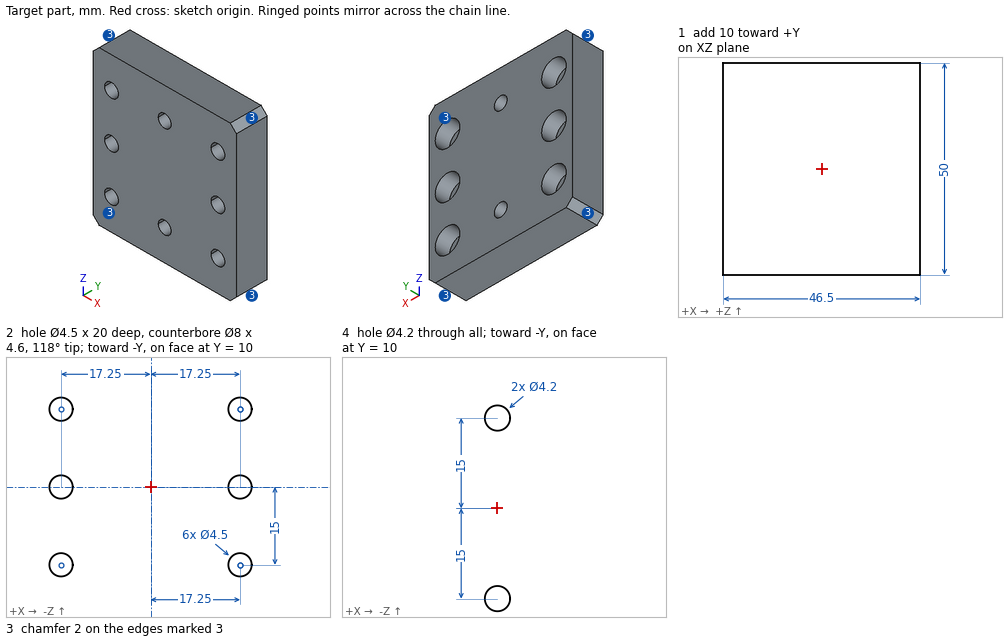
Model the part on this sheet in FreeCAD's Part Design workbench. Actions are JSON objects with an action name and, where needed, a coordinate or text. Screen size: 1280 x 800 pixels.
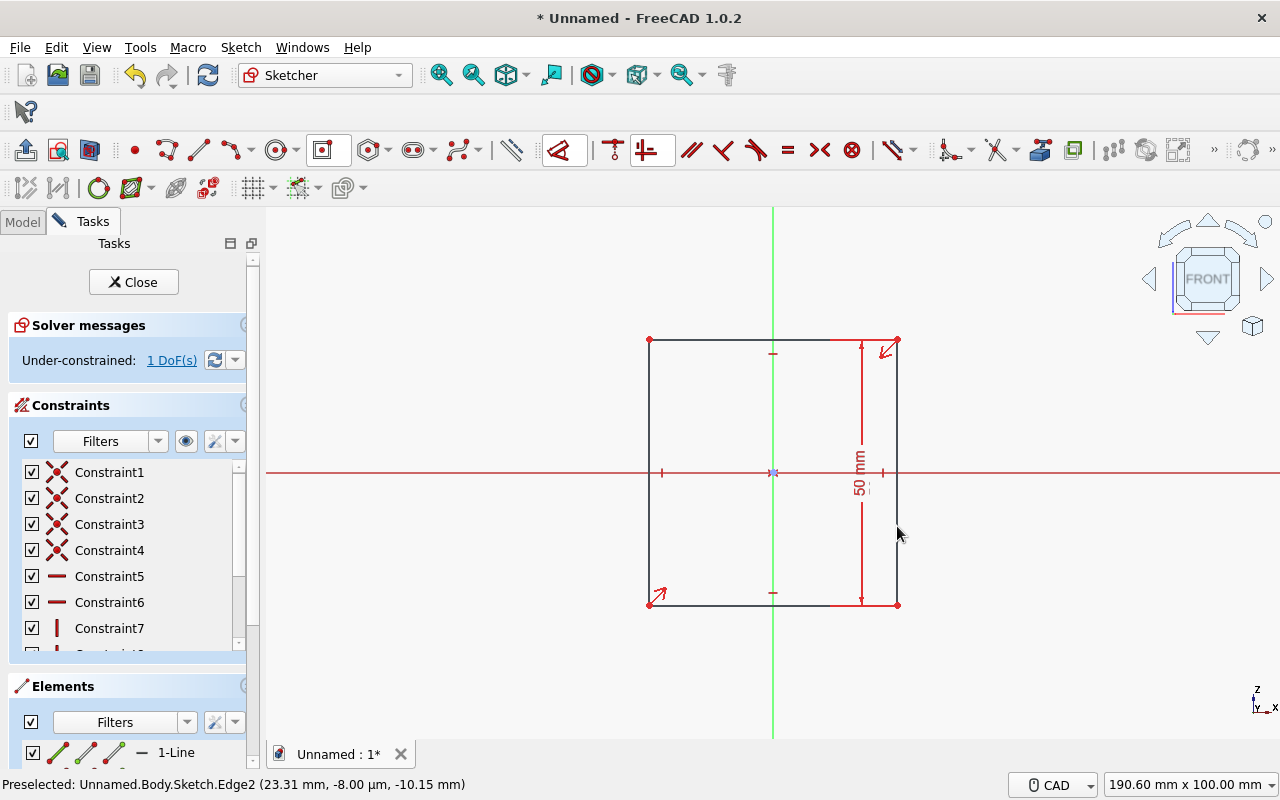
{"action": "left_click", "coordinate": [723, 606]}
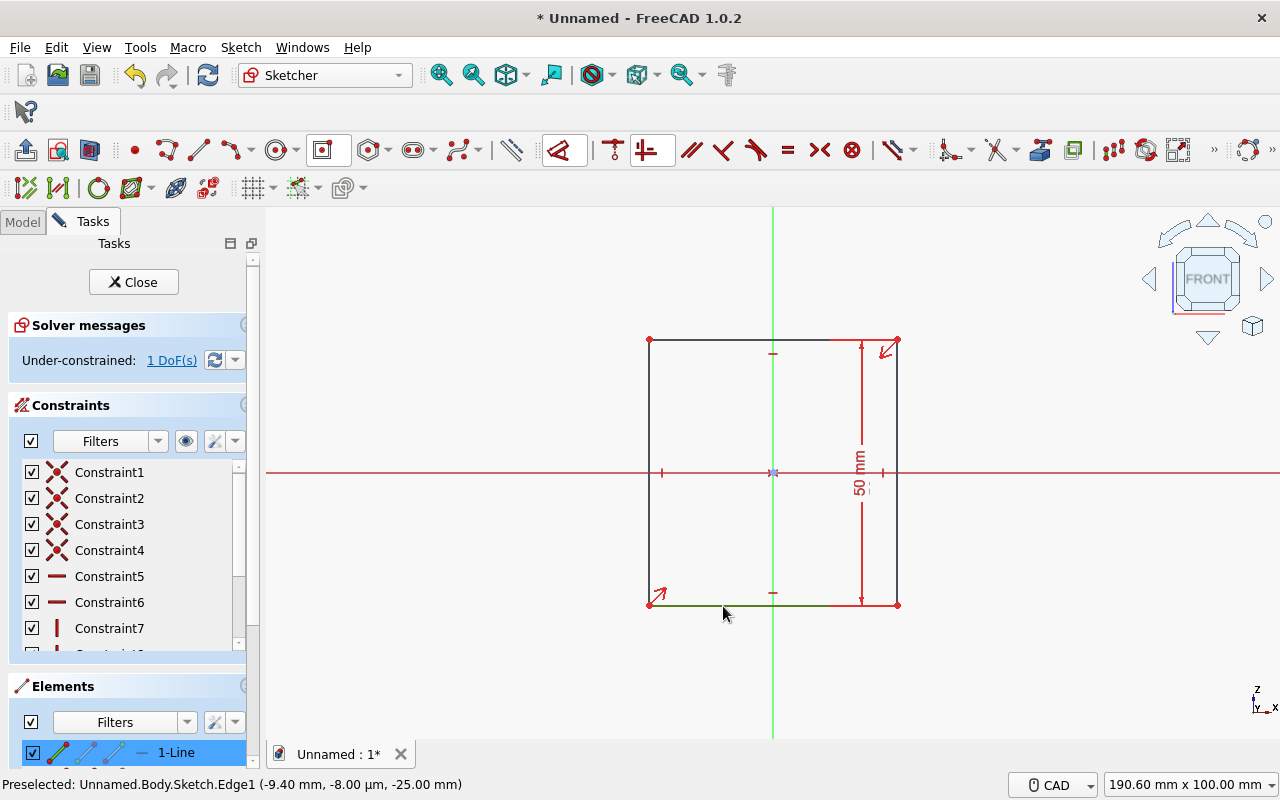
{"action": "left_click", "coordinate": [582, 150]}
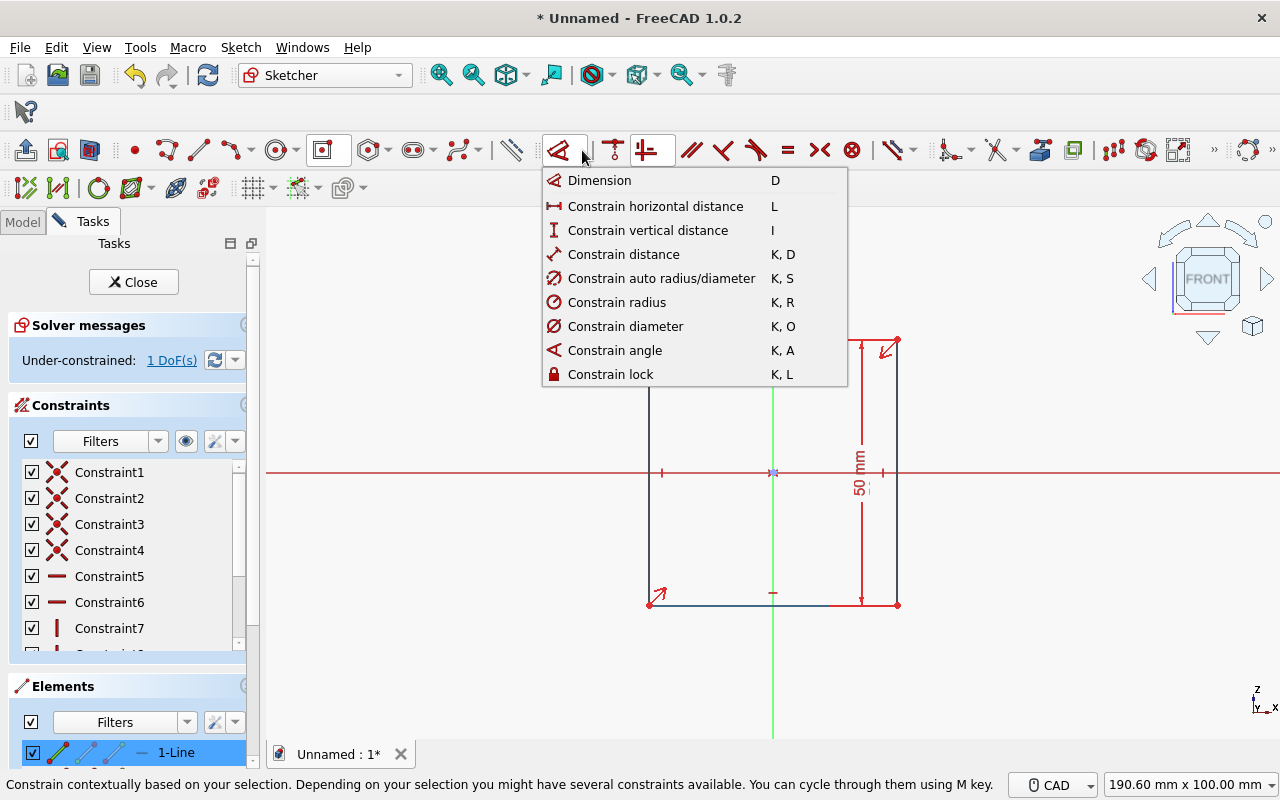
{"action": "left_click", "coordinate": [695, 206]}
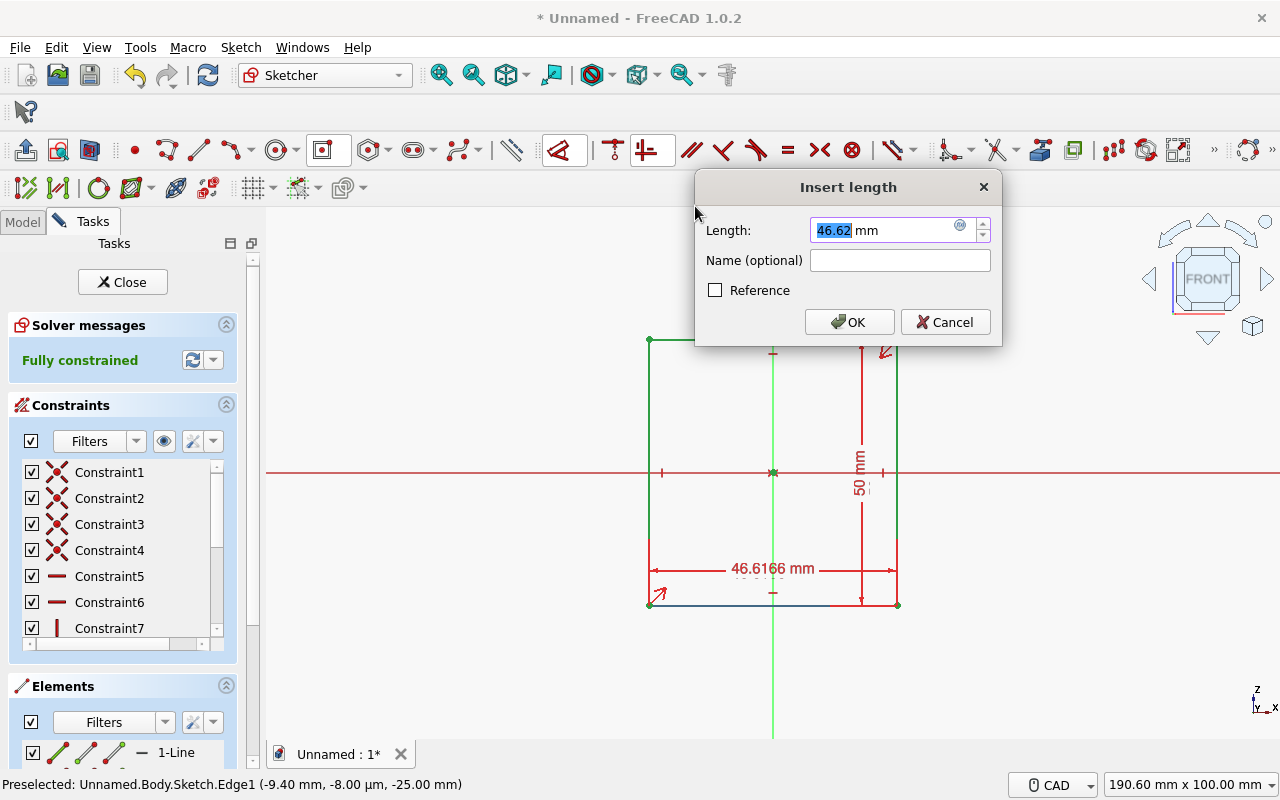
{"action": "type", "text": "46.5"}
{"action": "key", "text": "Return"}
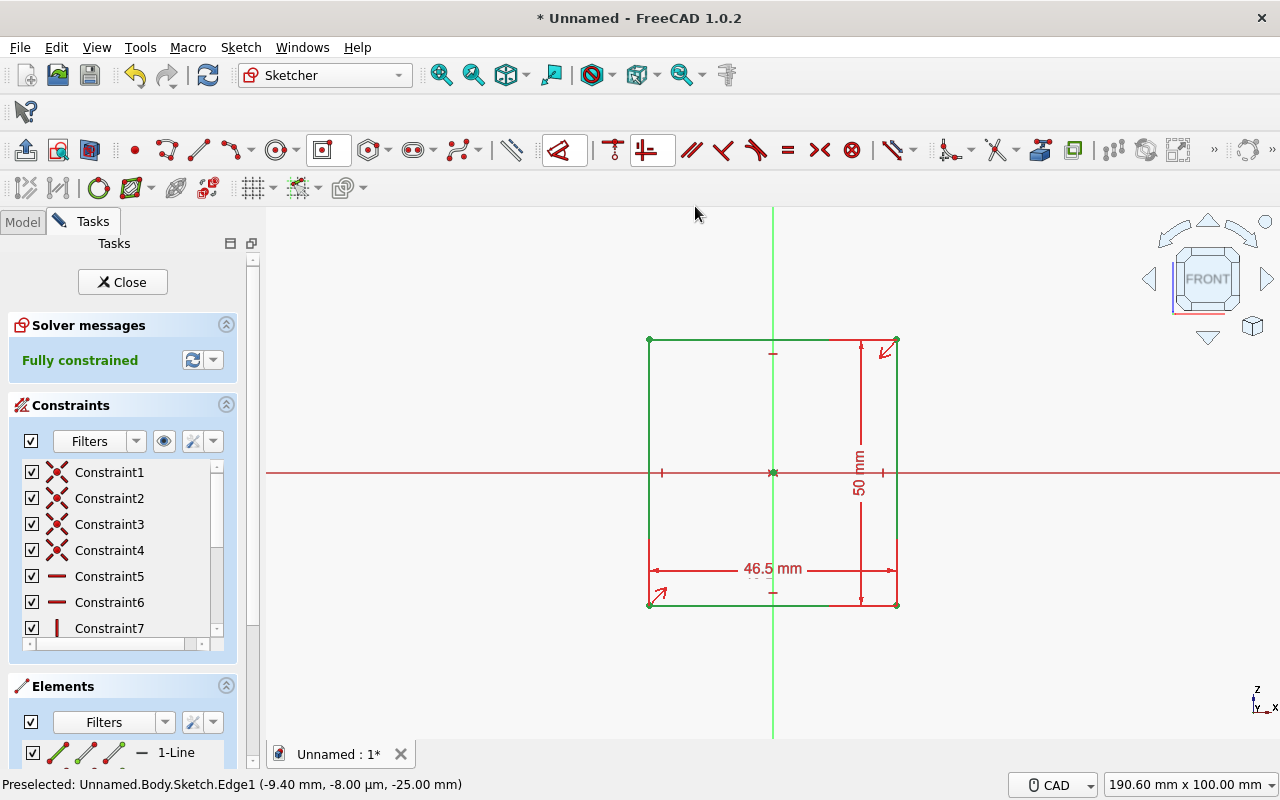
{"action": "left_click", "coordinate": [123, 282]}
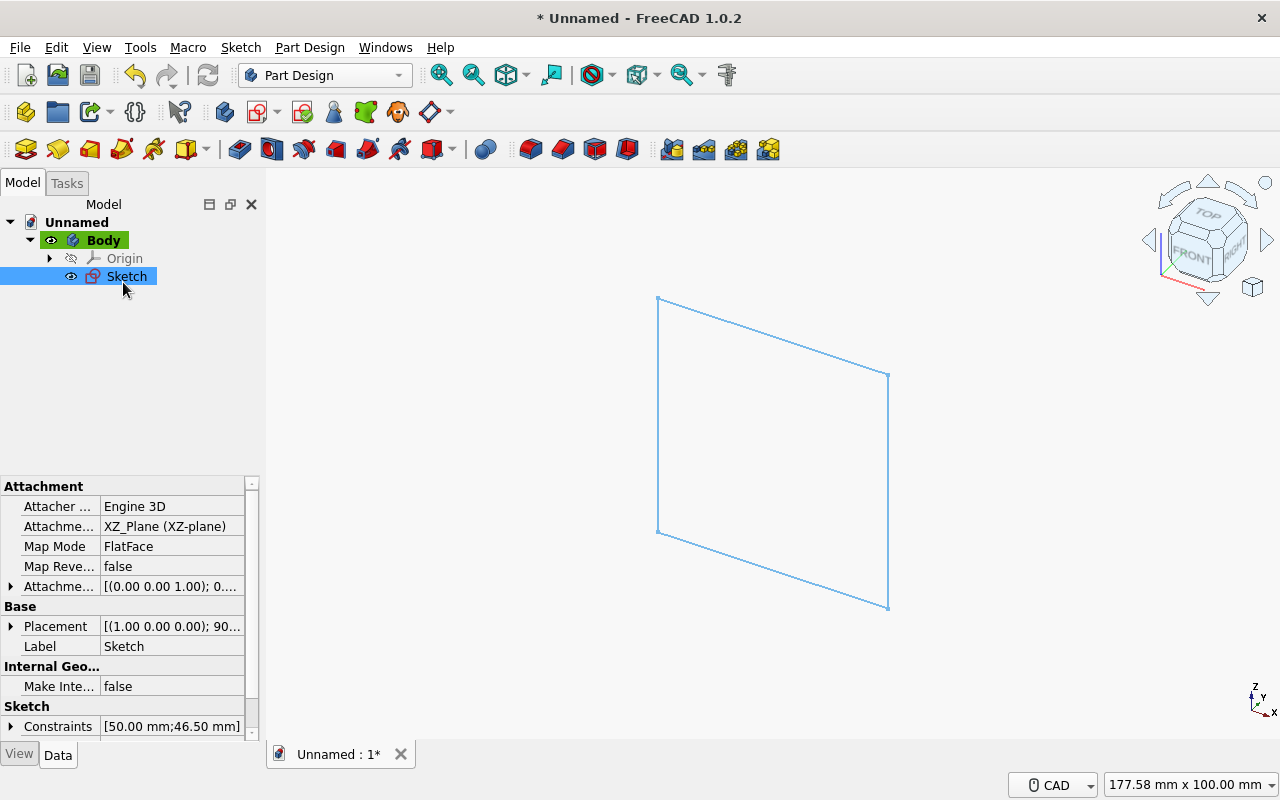
{"action": "left_click", "coordinate": [26, 150]}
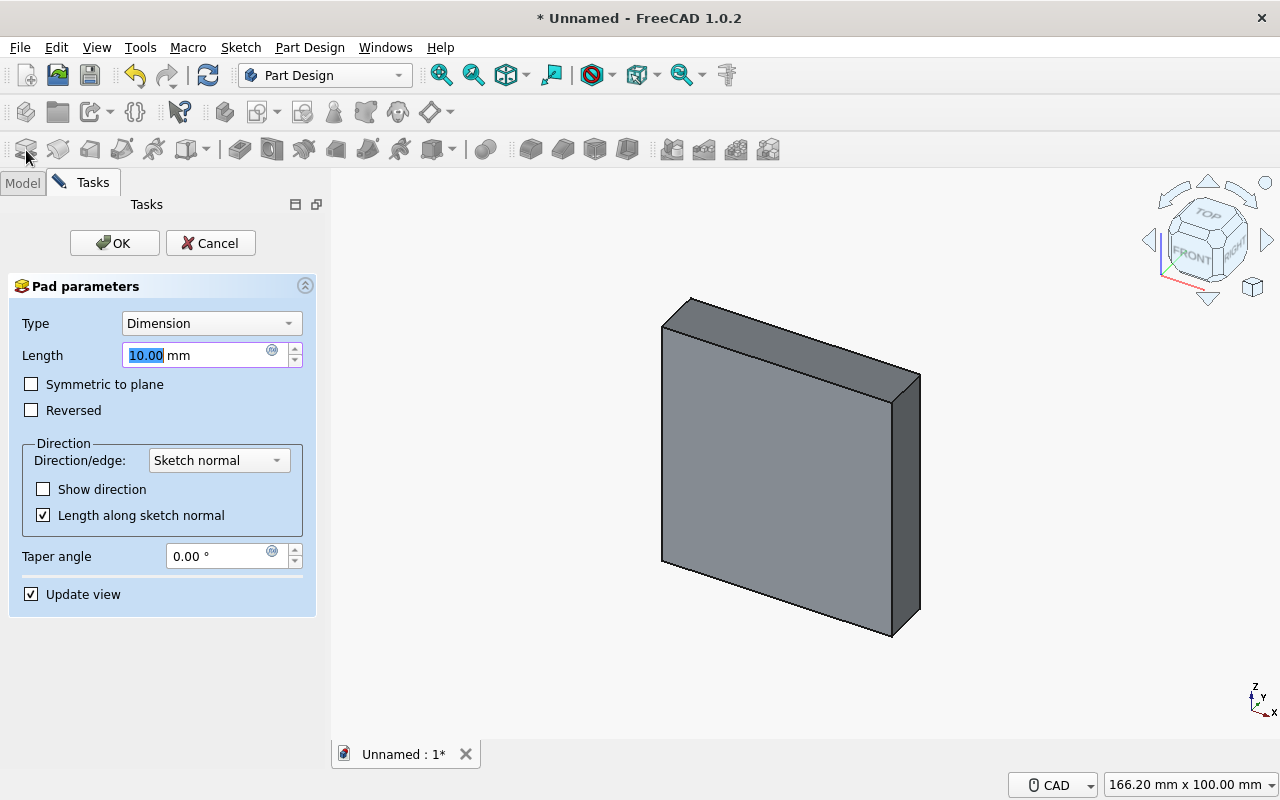
{"action": "type", "text": "10"}
{"action": "key", "text": "Tab"}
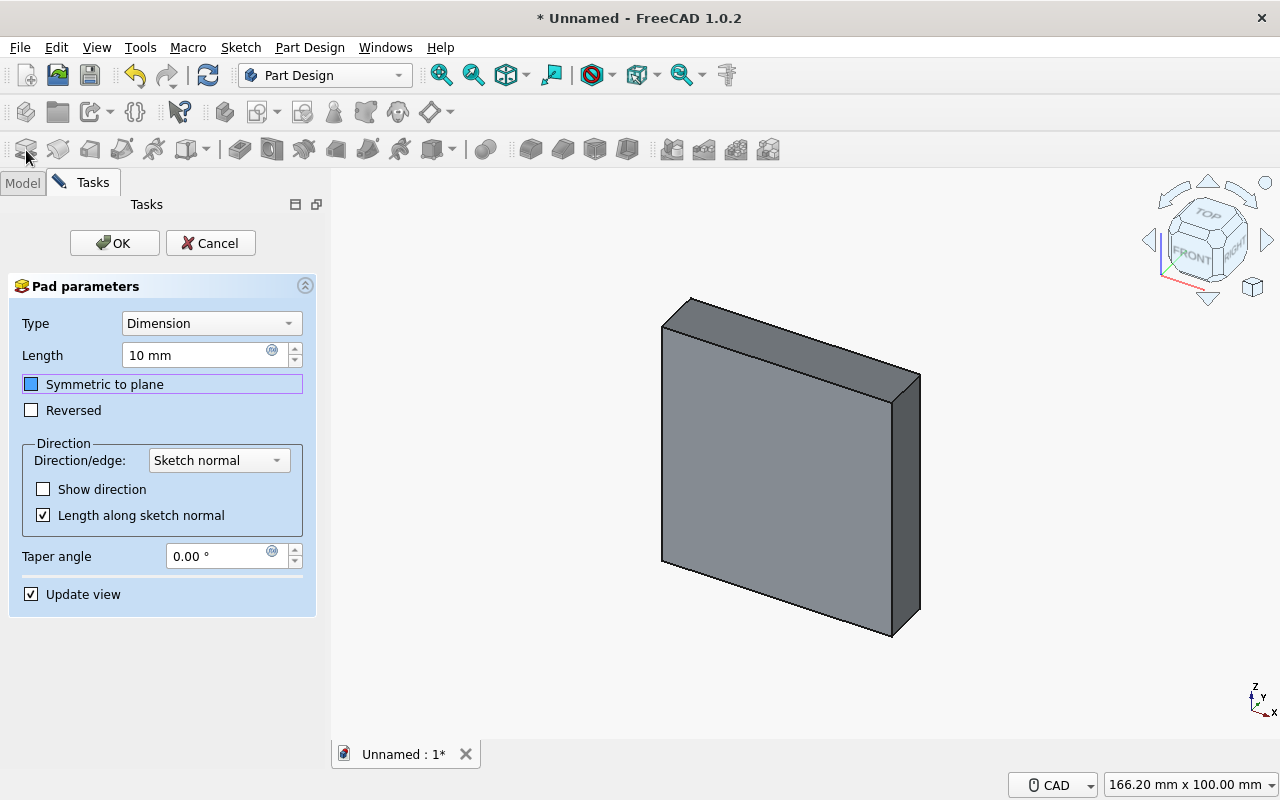
{"action": "left_click", "coordinate": [30, 410]}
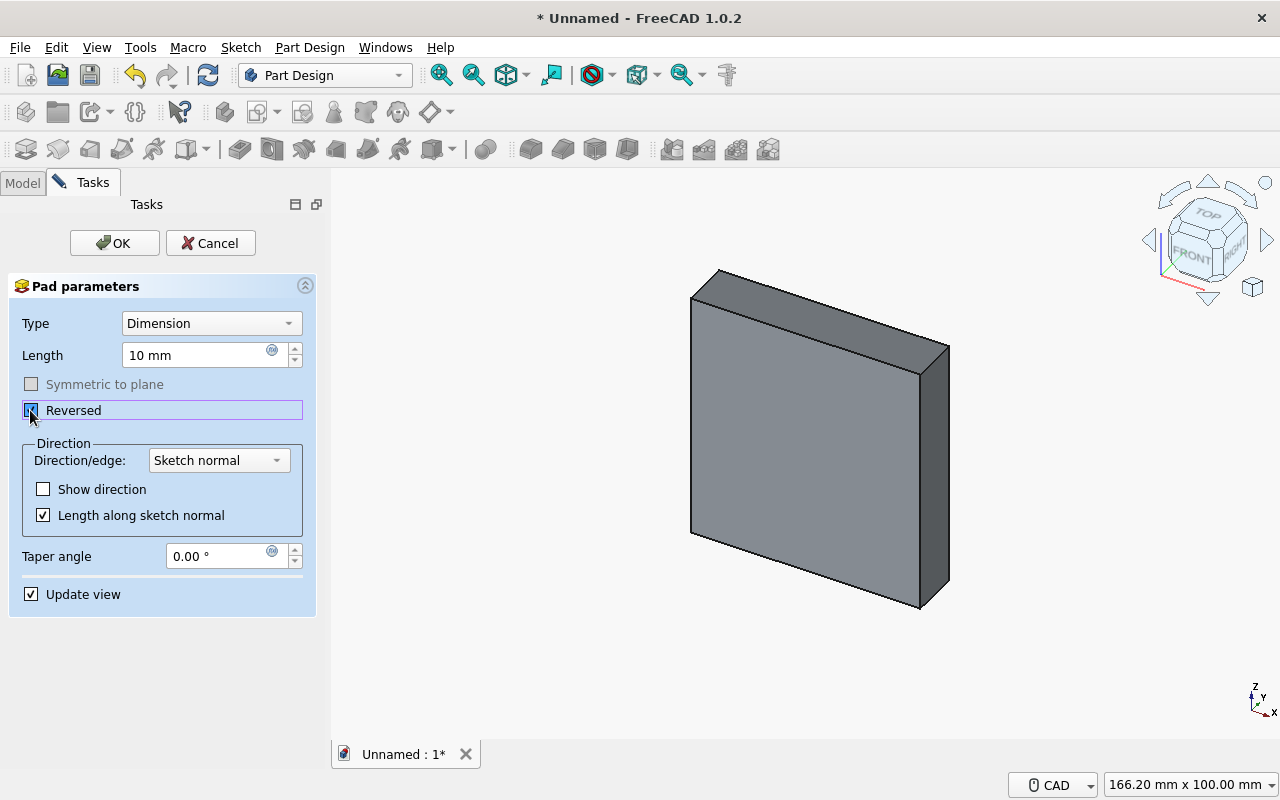
{"action": "left_click", "coordinate": [115, 243]}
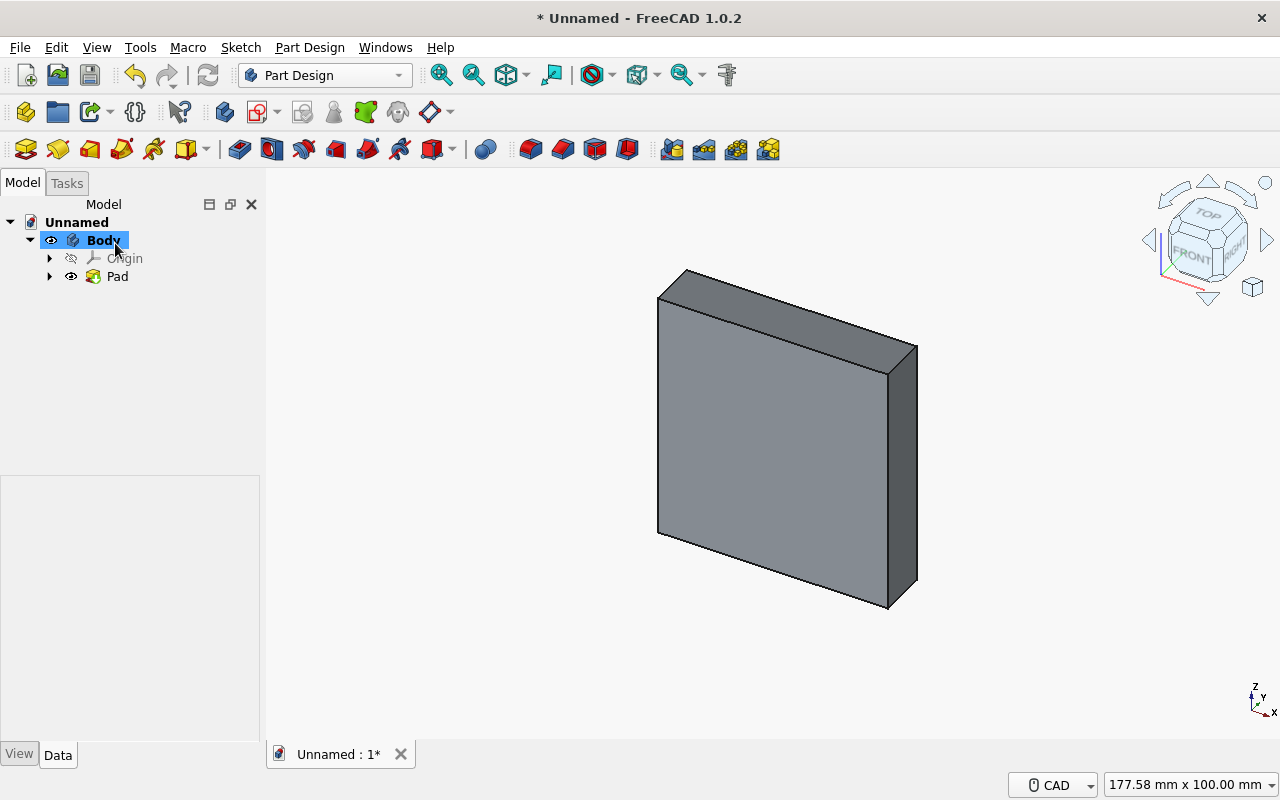
{"action": "key", "text": "4"}